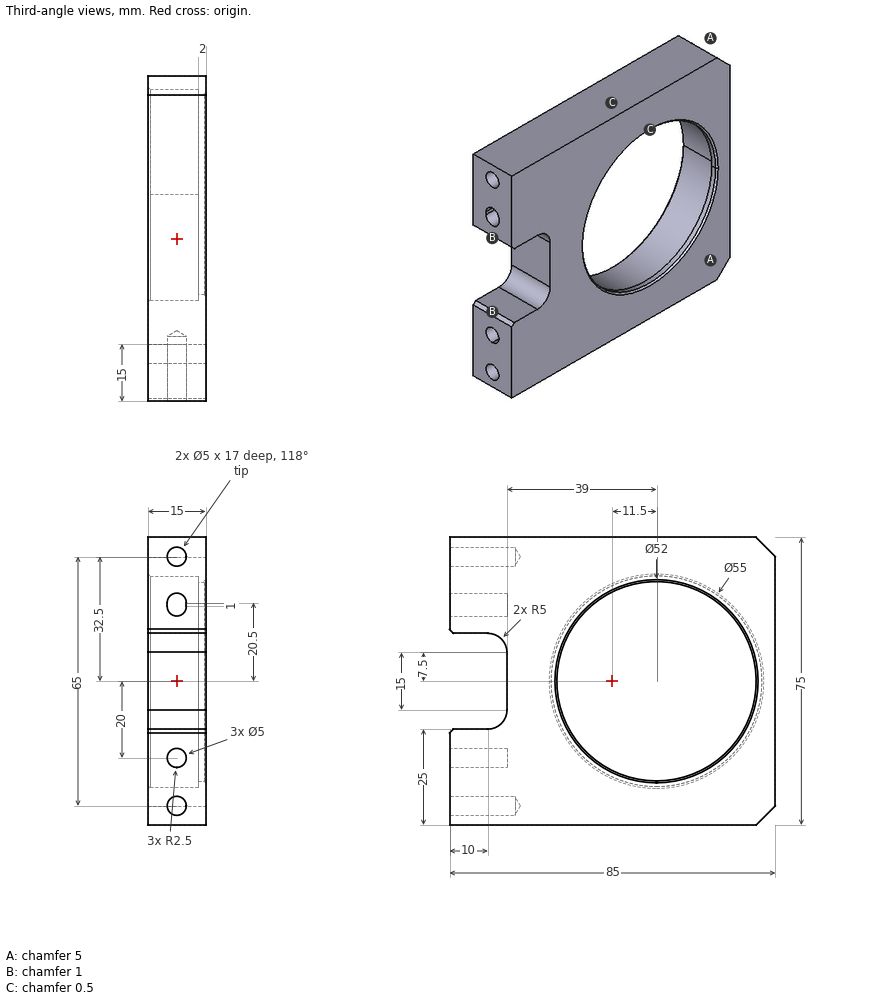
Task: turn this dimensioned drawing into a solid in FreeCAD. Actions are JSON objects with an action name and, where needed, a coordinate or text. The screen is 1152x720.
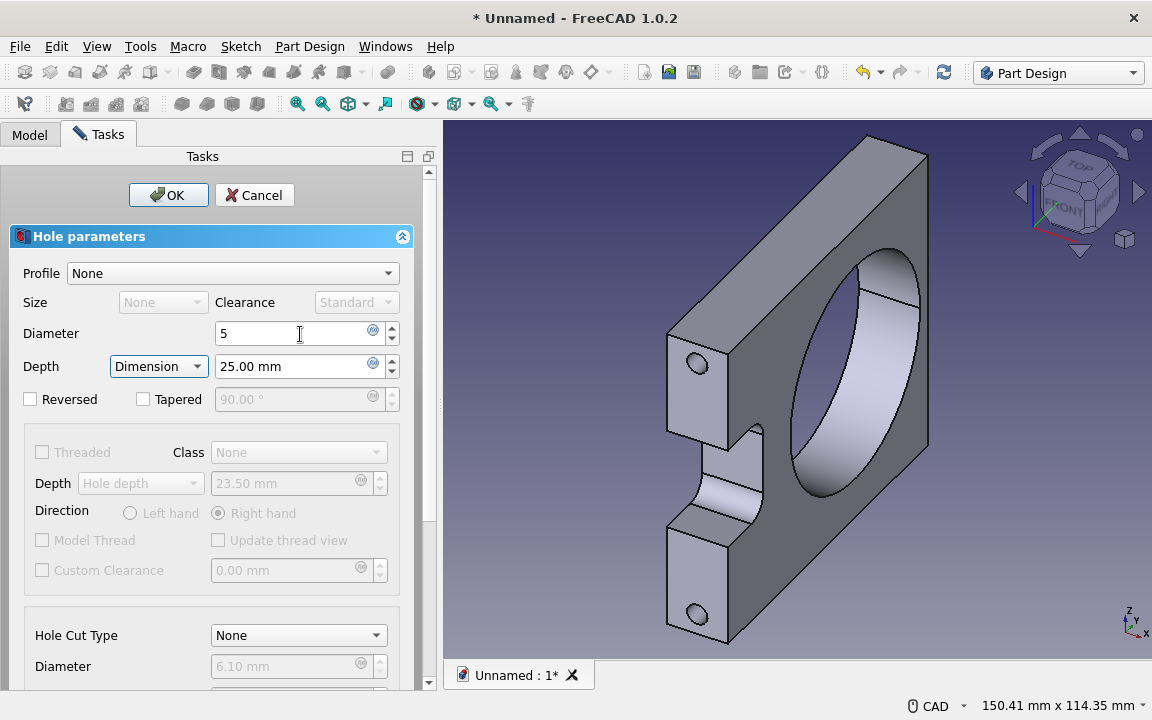
{"action": "triple_click", "coordinate": [300, 366]}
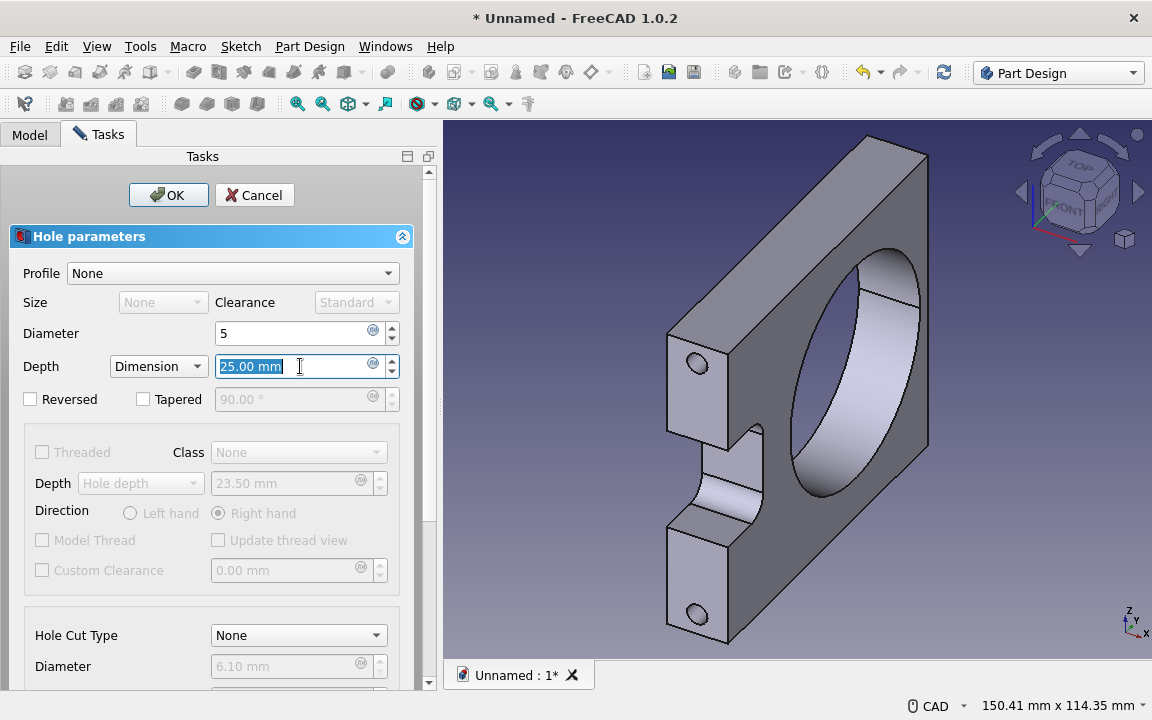
{"action": "type", "text": "17"}
{"action": "key", "text": "Tab"}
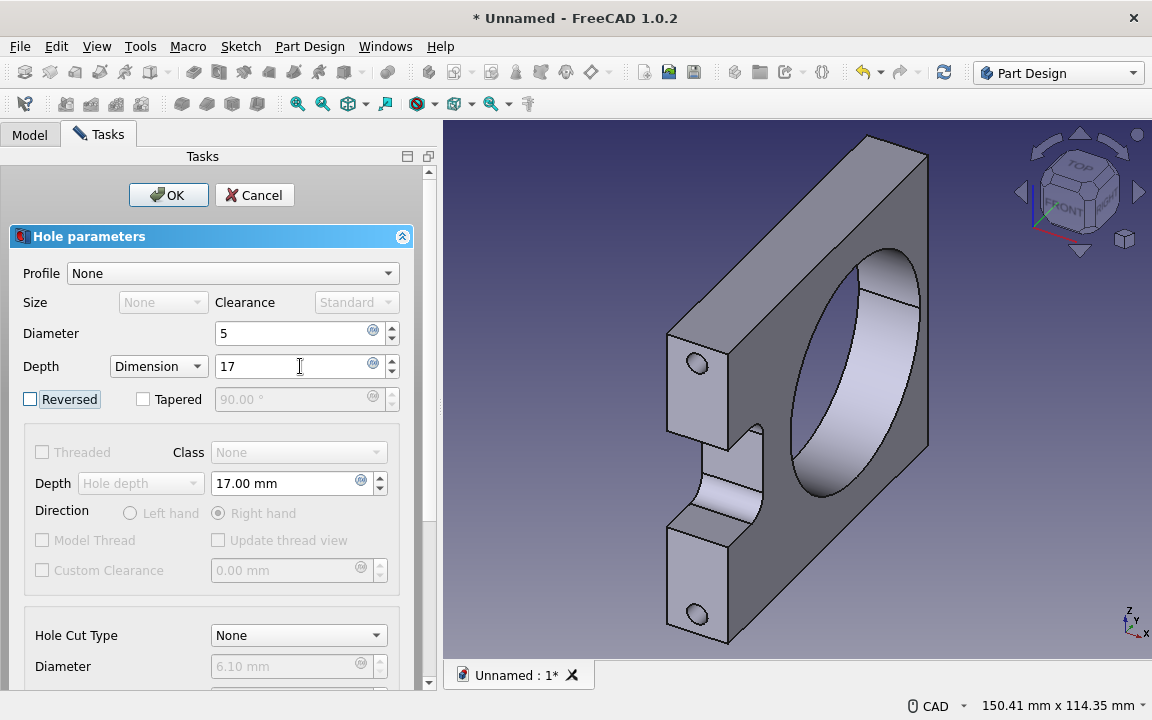
{"action": "left_click", "coordinate": [169, 195]}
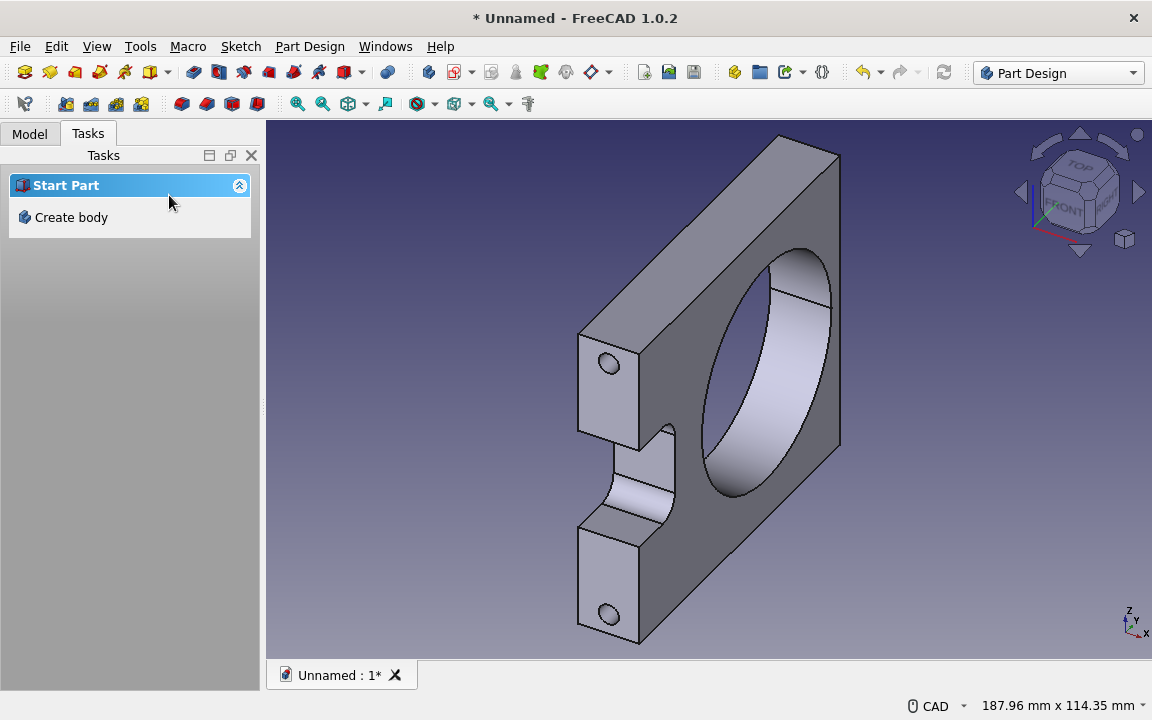
{"action": "left_click", "coordinate": [30, 134]}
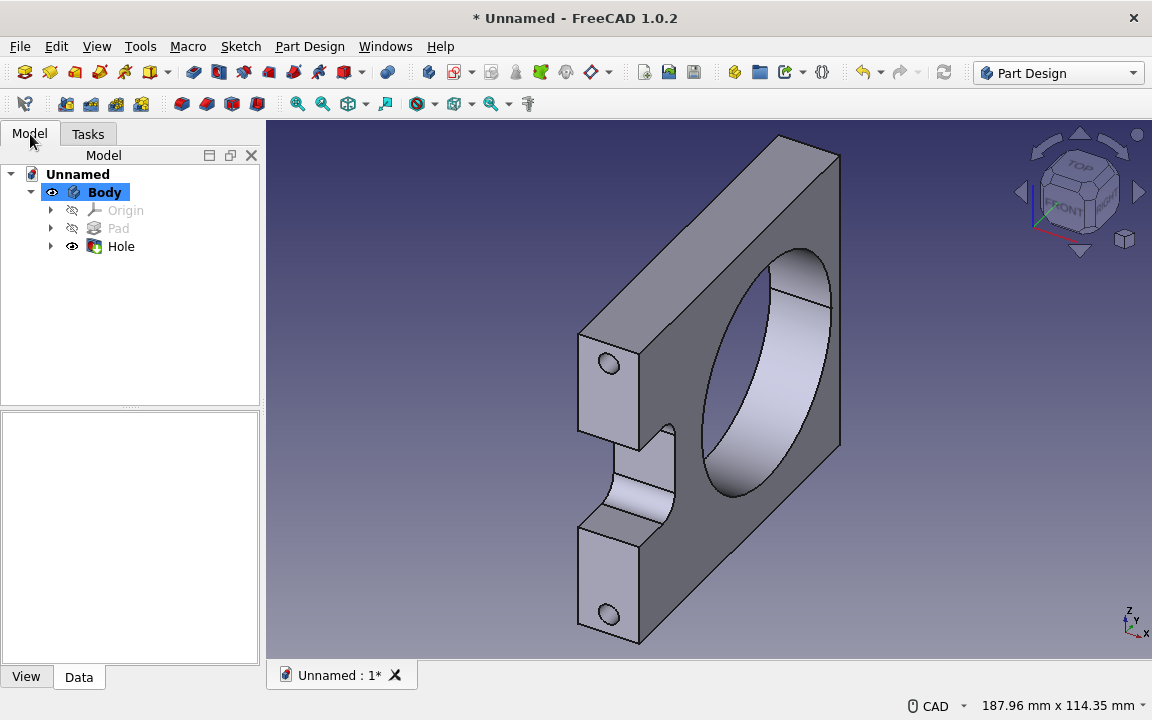
{"action": "left_click", "coordinate": [51, 210]}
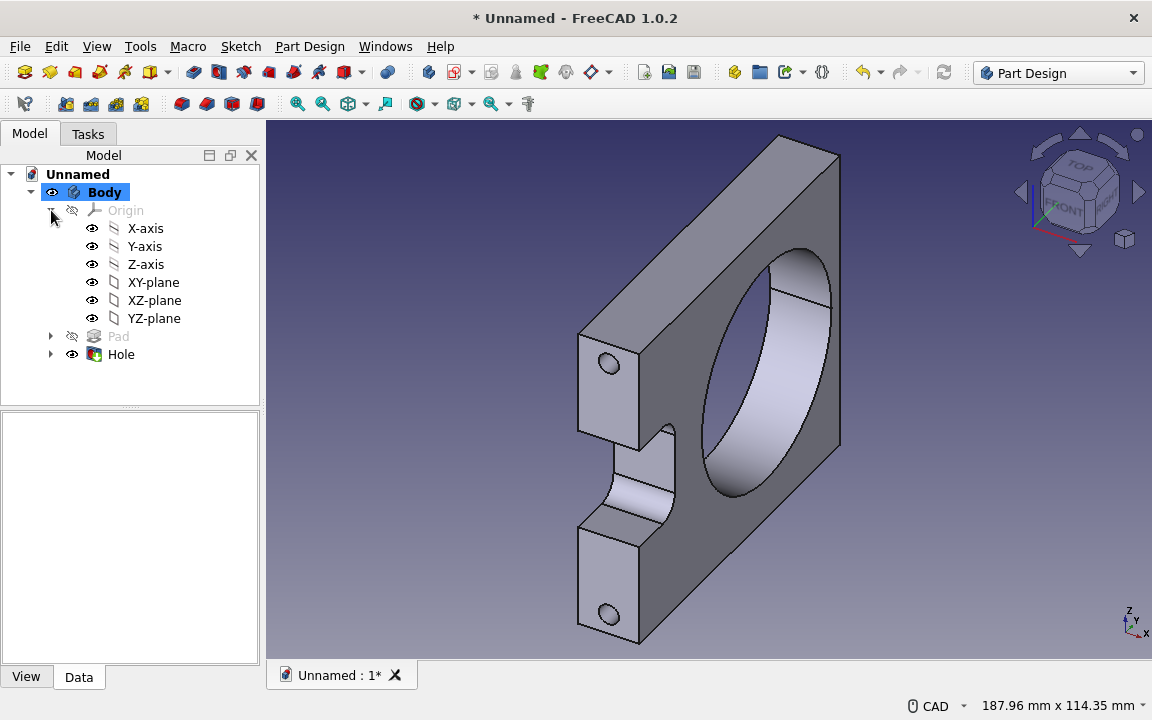
{"action": "left_click", "coordinate": [137, 318]}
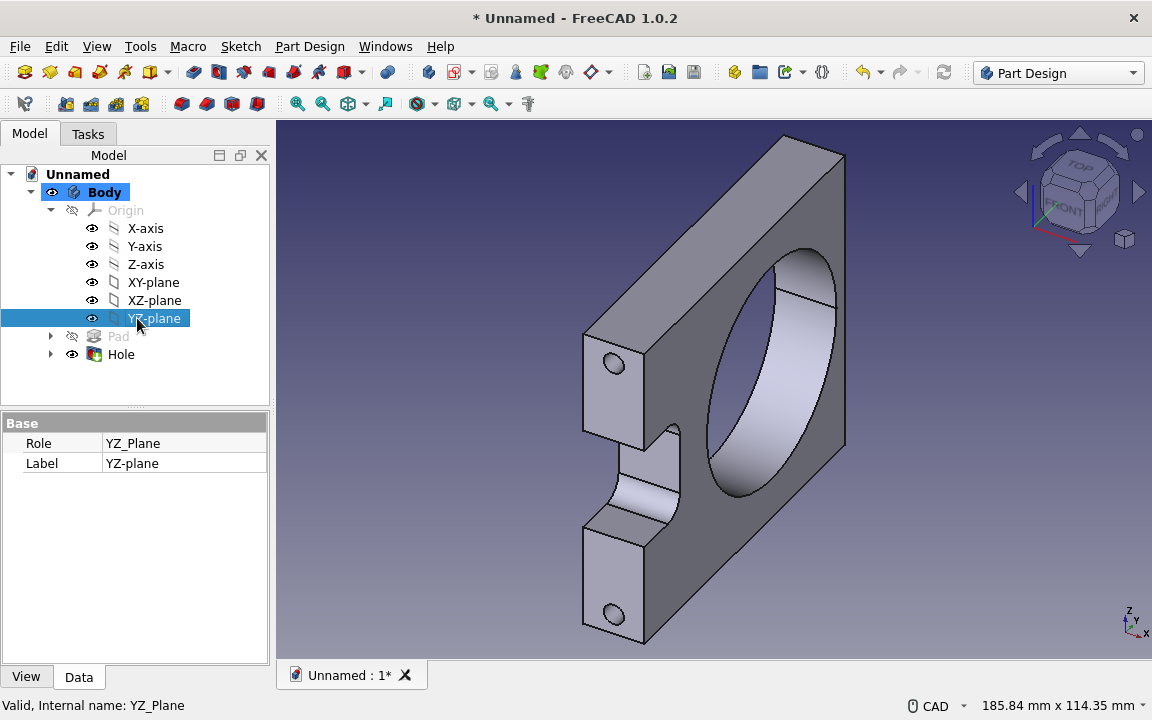
{"action": "left_click", "coordinate": [590, 72]}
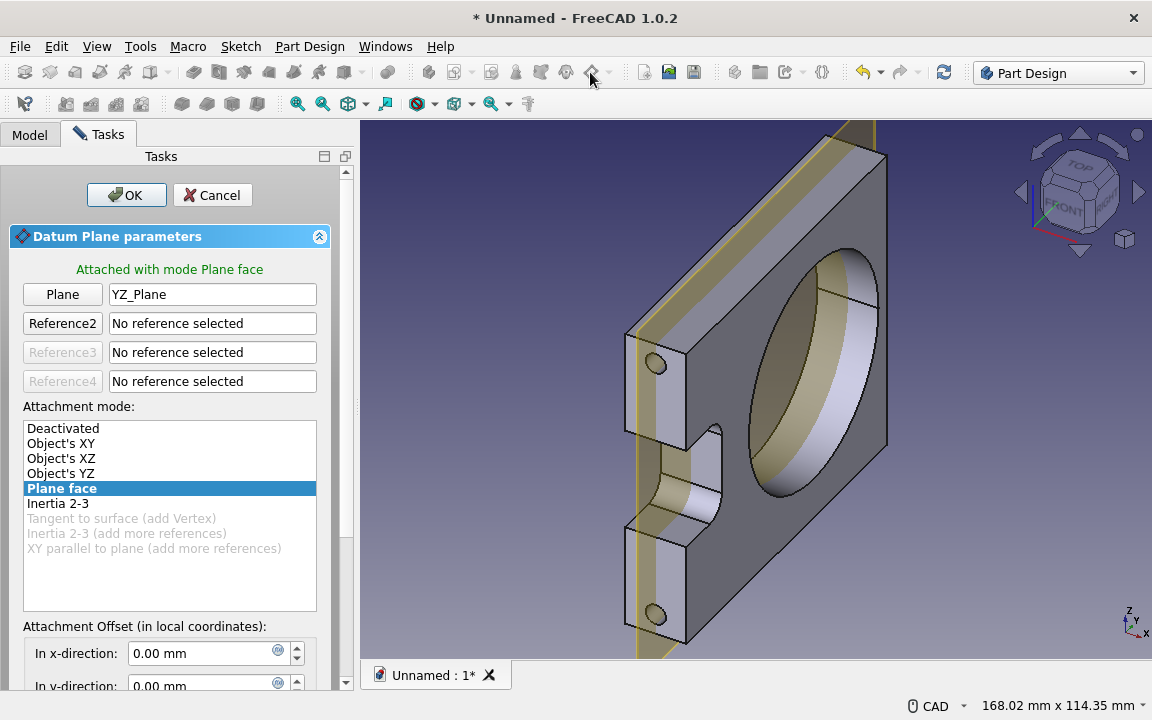
{"action": "scroll", "coordinate": [346, 428], "scroll_direction": "down", "scroll_amount": 2}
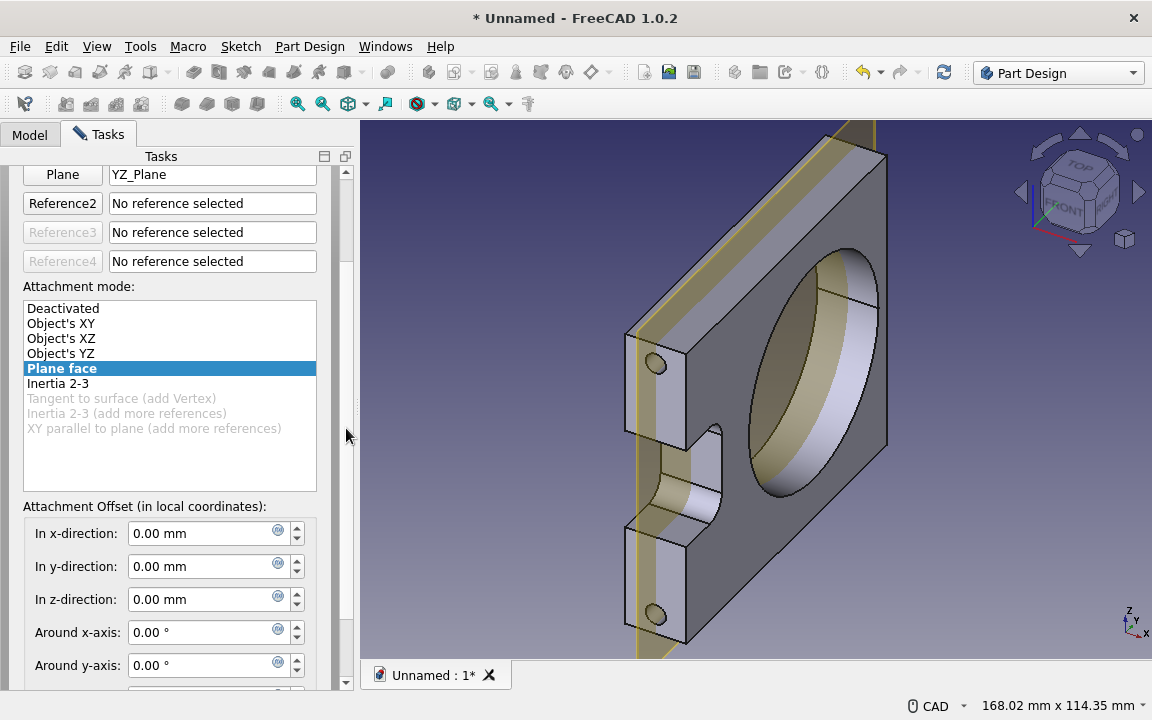
{"action": "triple_click", "coordinate": [210, 600]}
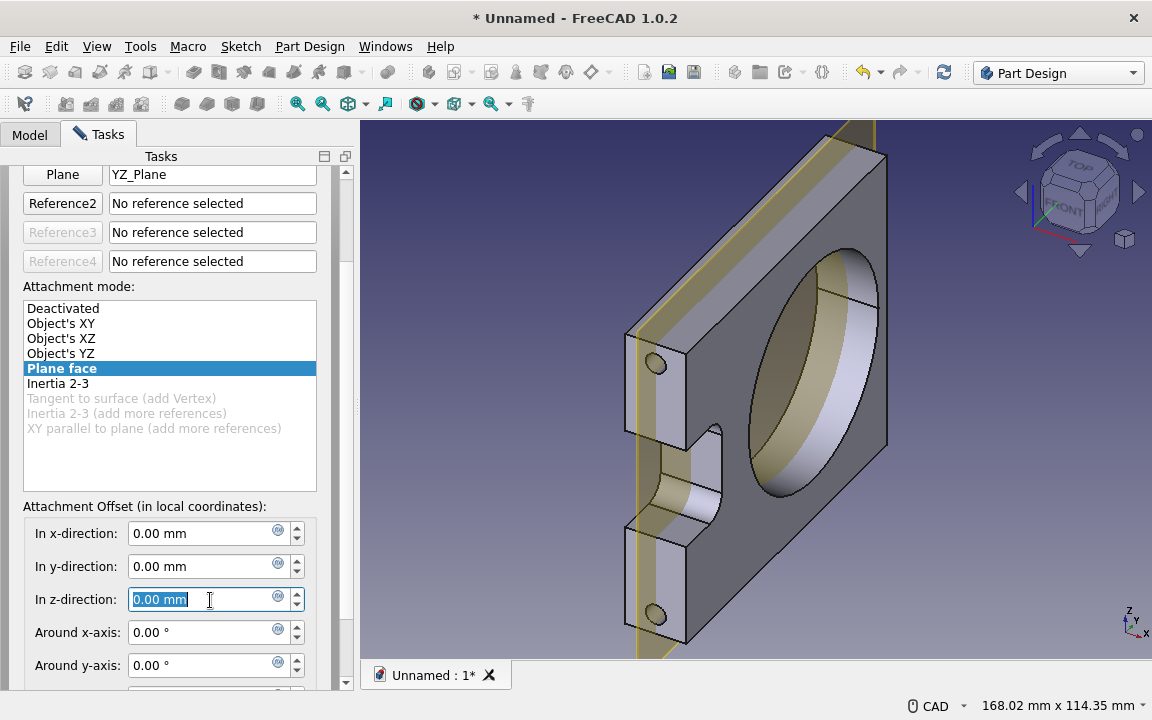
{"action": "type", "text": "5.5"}
{"action": "key", "text": "Tab"}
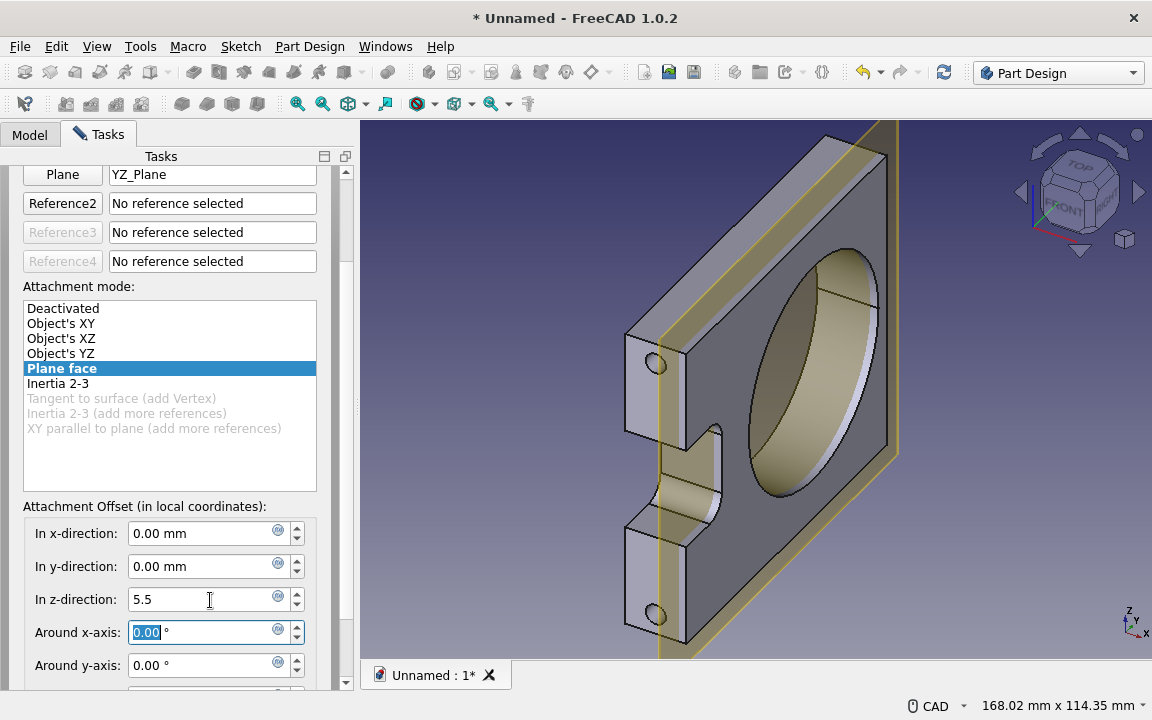
{"action": "scroll", "coordinate": [346, 428], "scroll_direction": "up", "scroll_amount": 3}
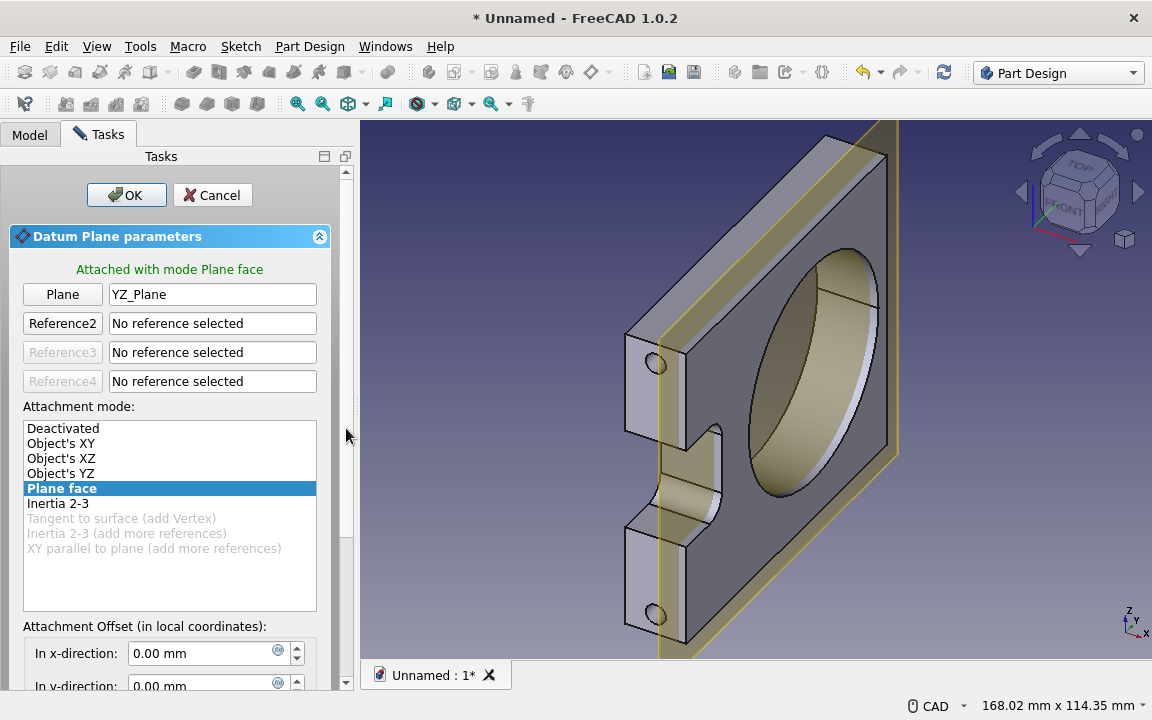
{"action": "left_click", "coordinate": [127, 195]}